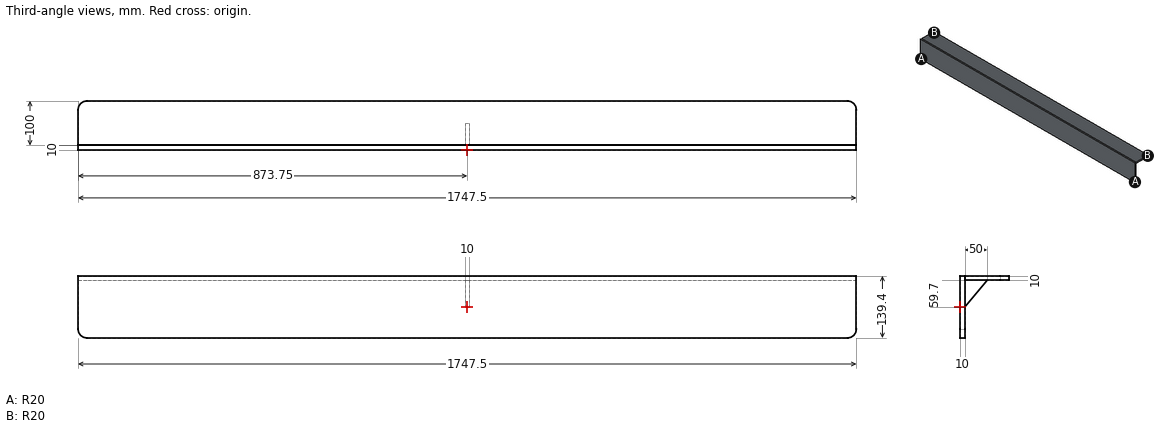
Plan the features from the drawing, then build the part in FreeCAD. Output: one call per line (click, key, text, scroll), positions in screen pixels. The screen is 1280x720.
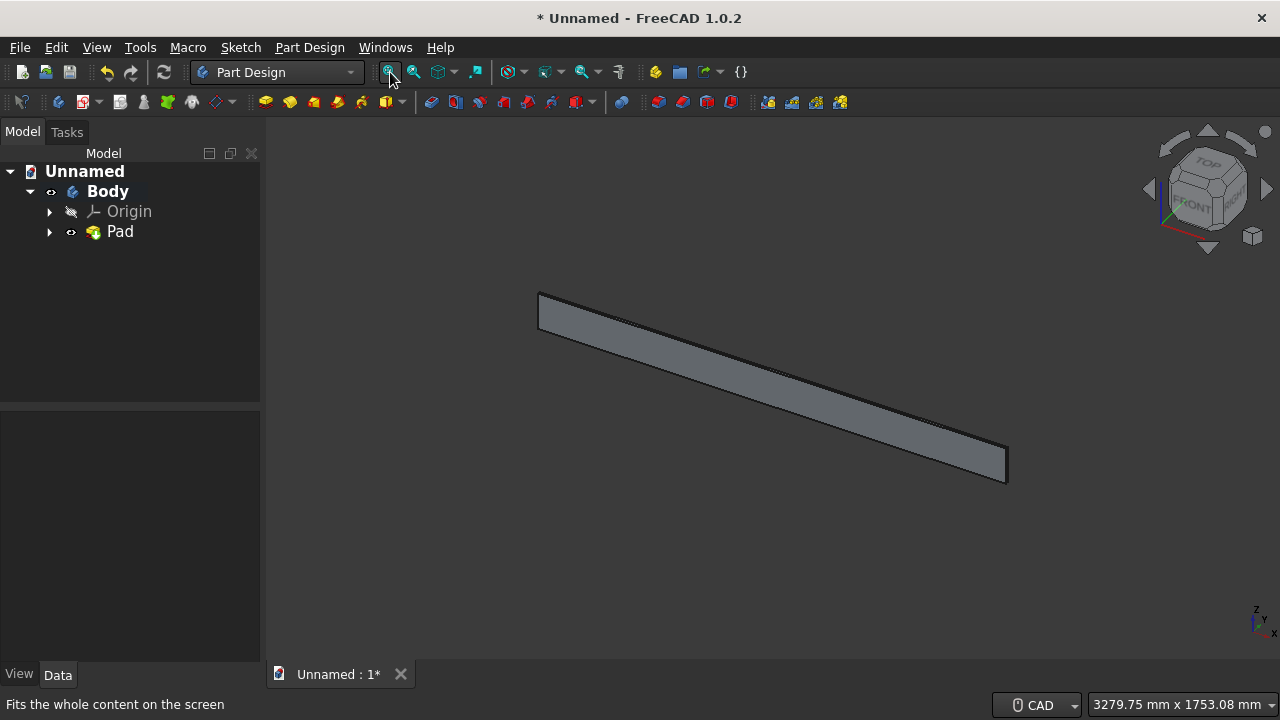
key(0)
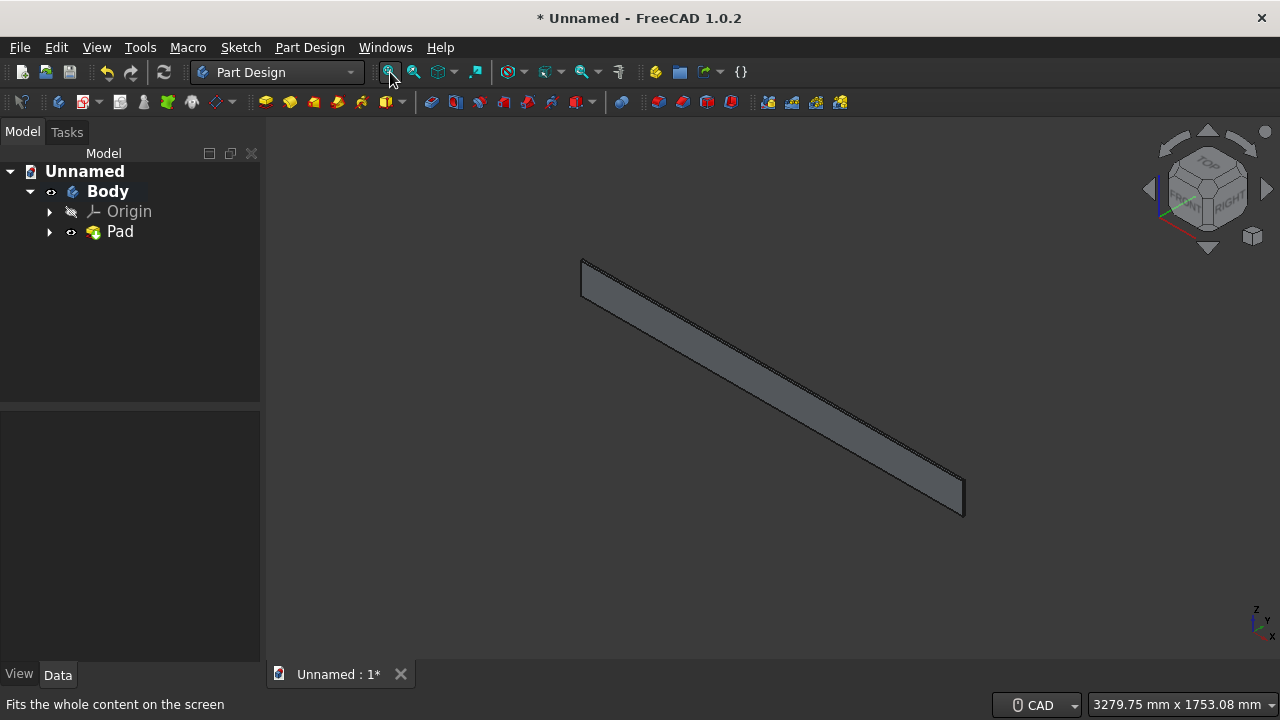
scroll(582, 294, up, 13)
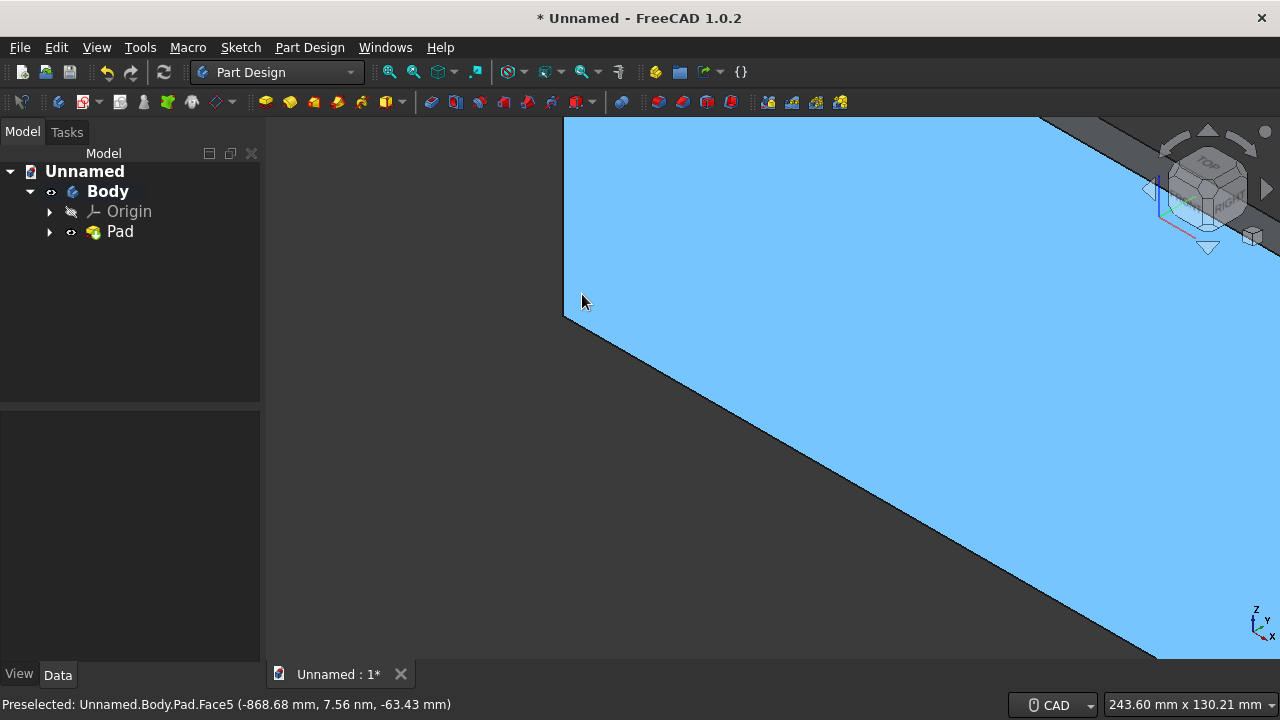
click(390, 72)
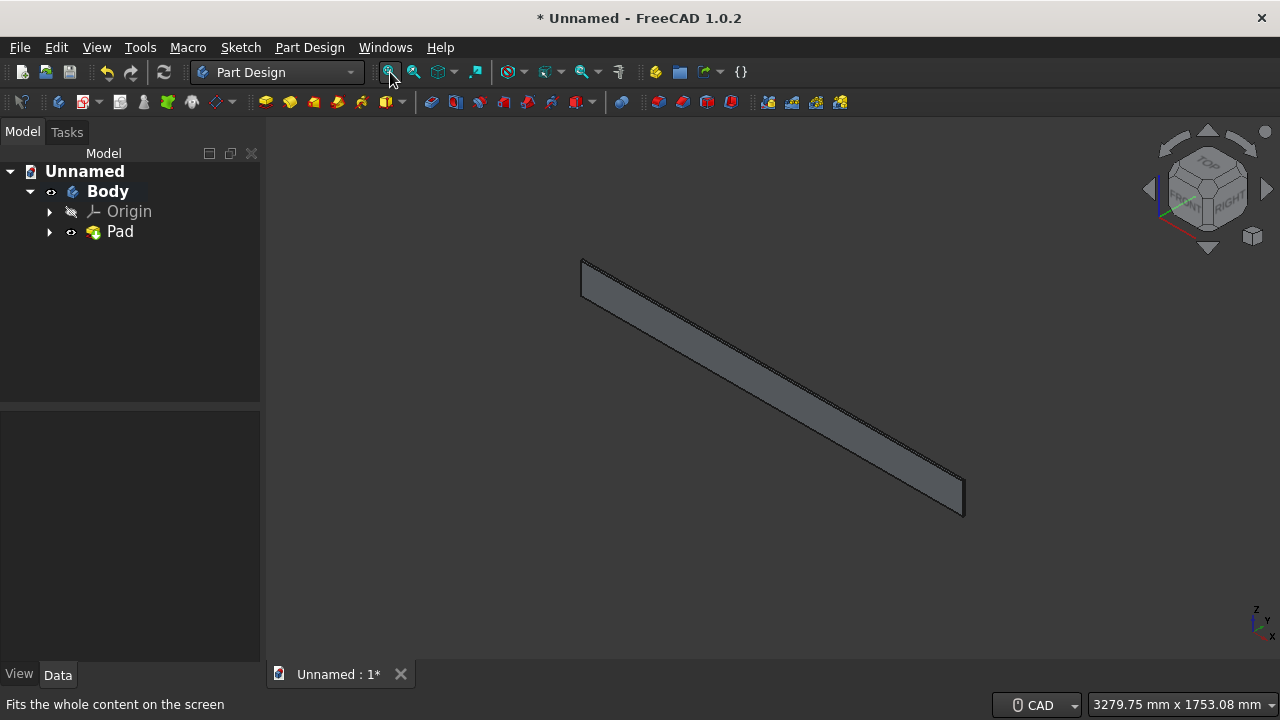
key(2)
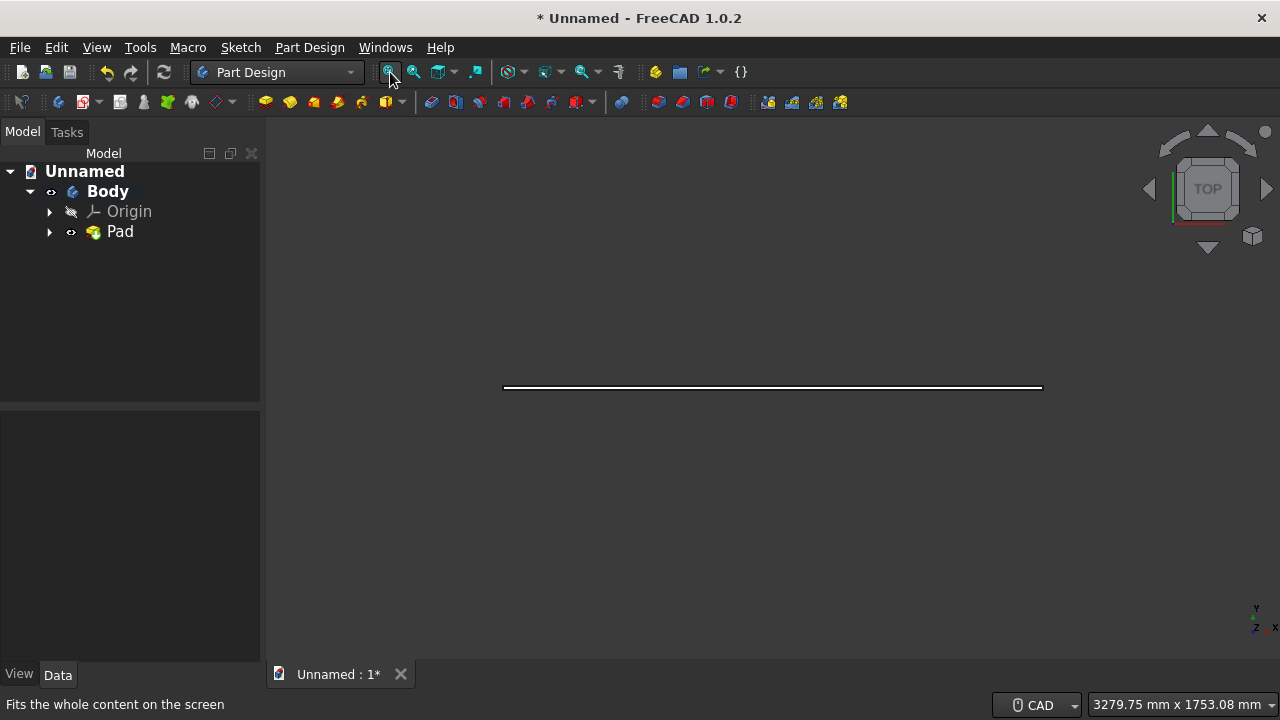
scroll(503, 387, up, 13)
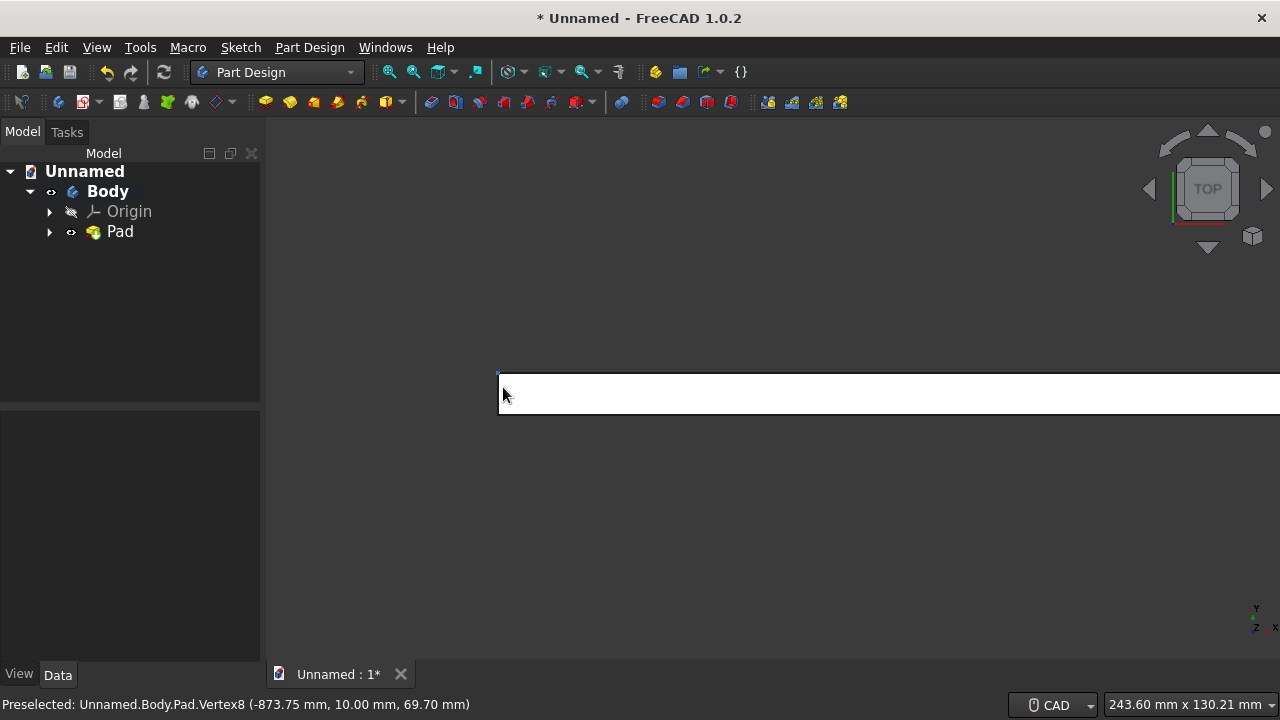
click(390, 72)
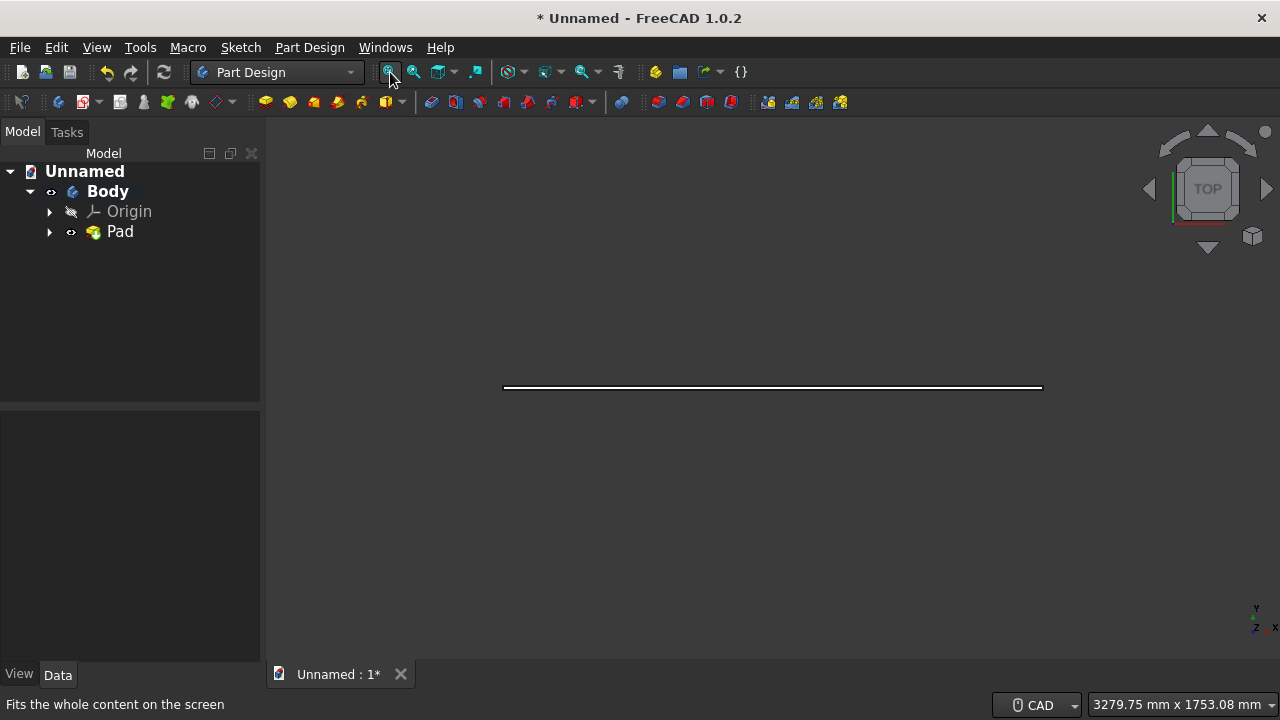
key(1)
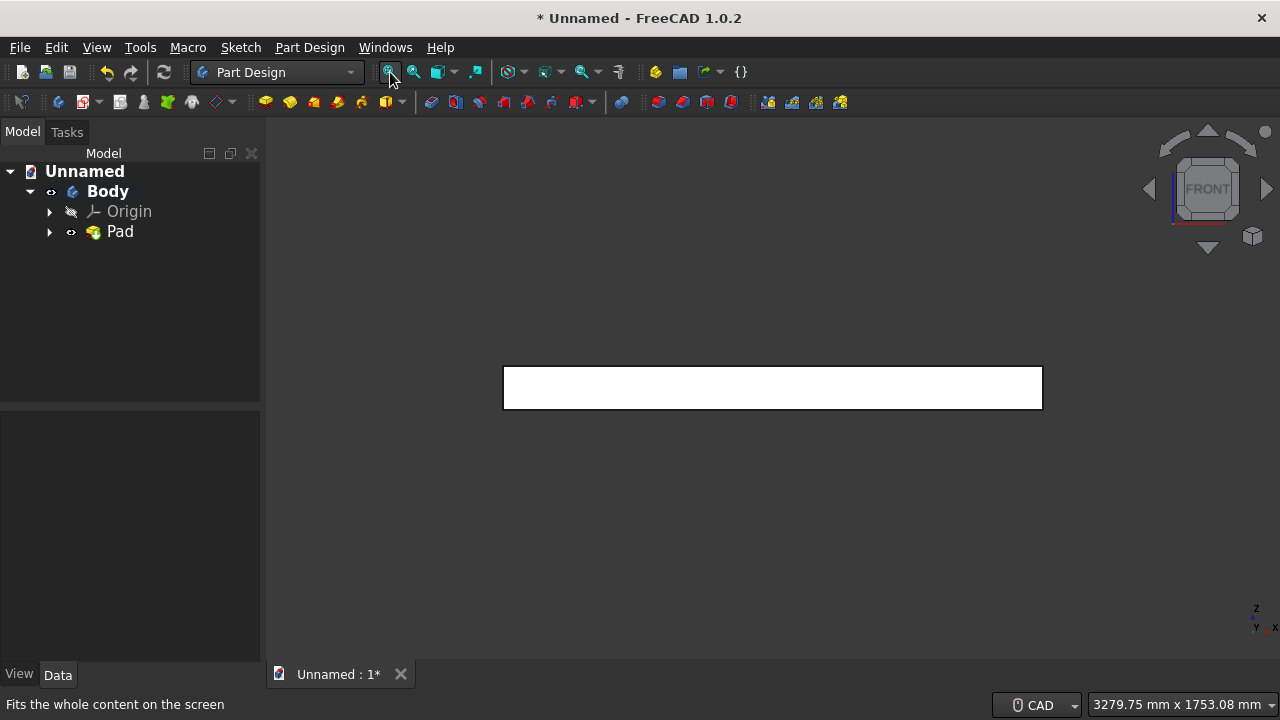
scroll(503, 409, up, 13)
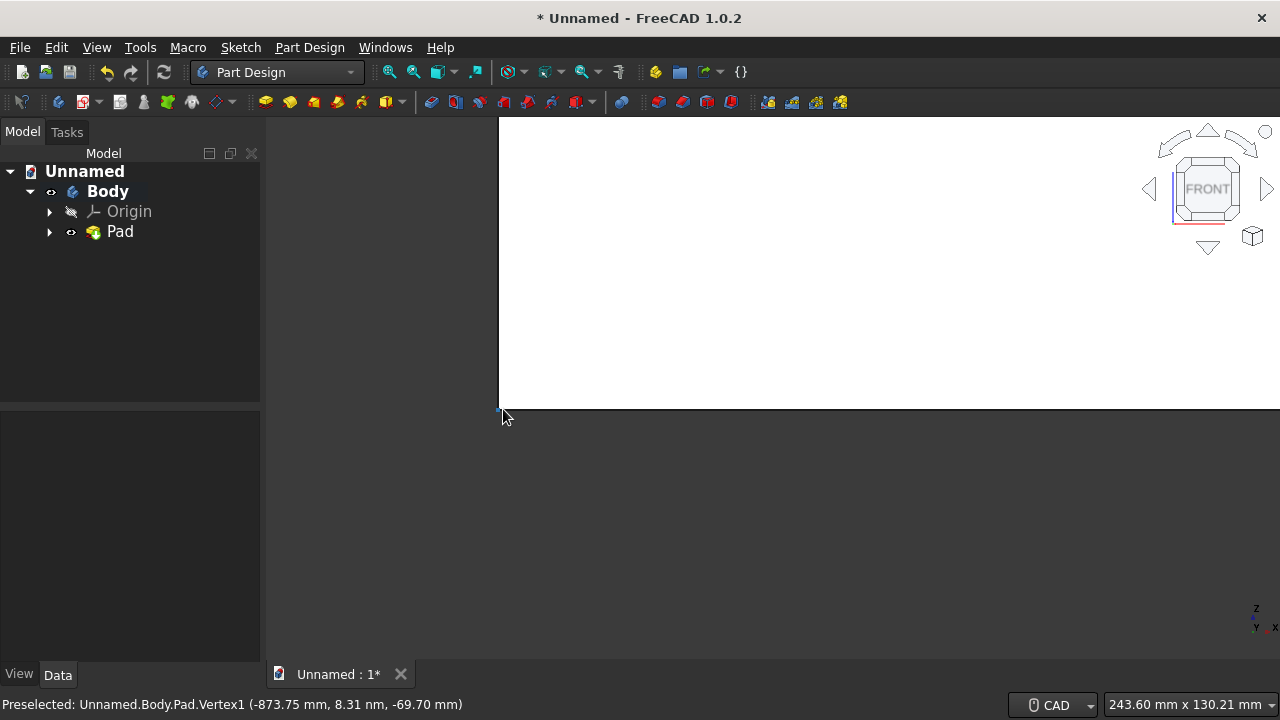
click(390, 72)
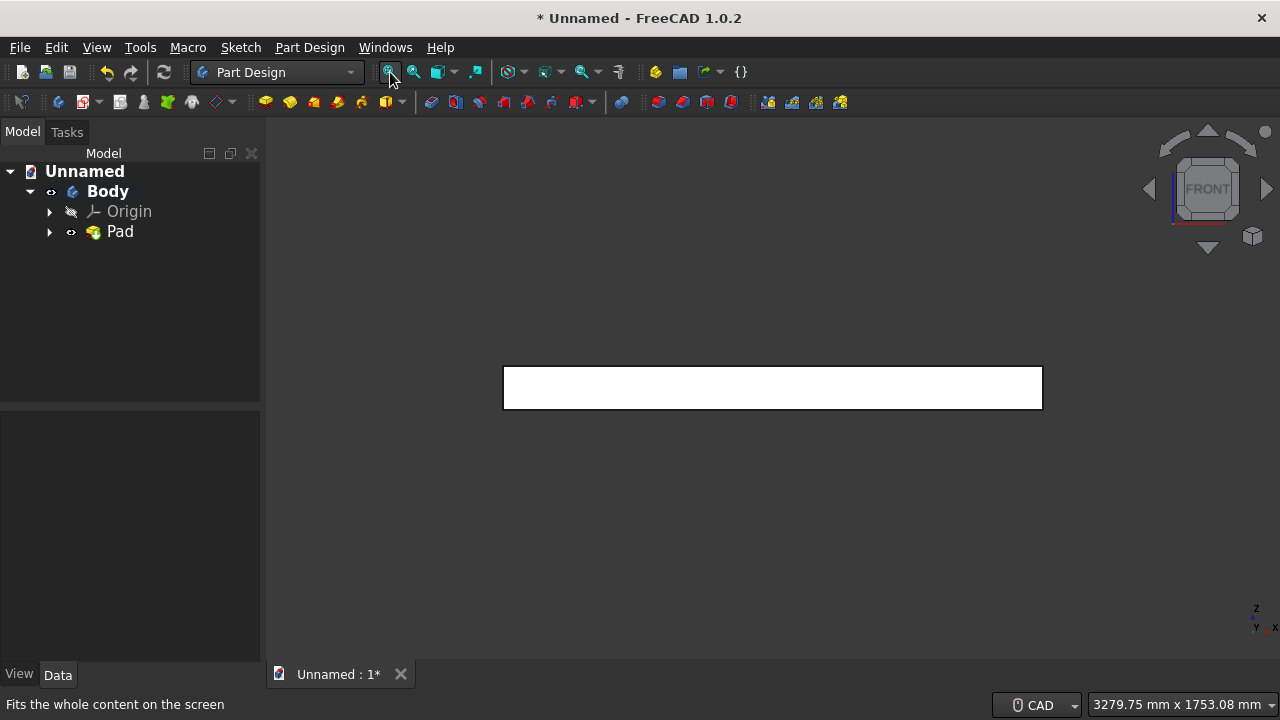
key(3)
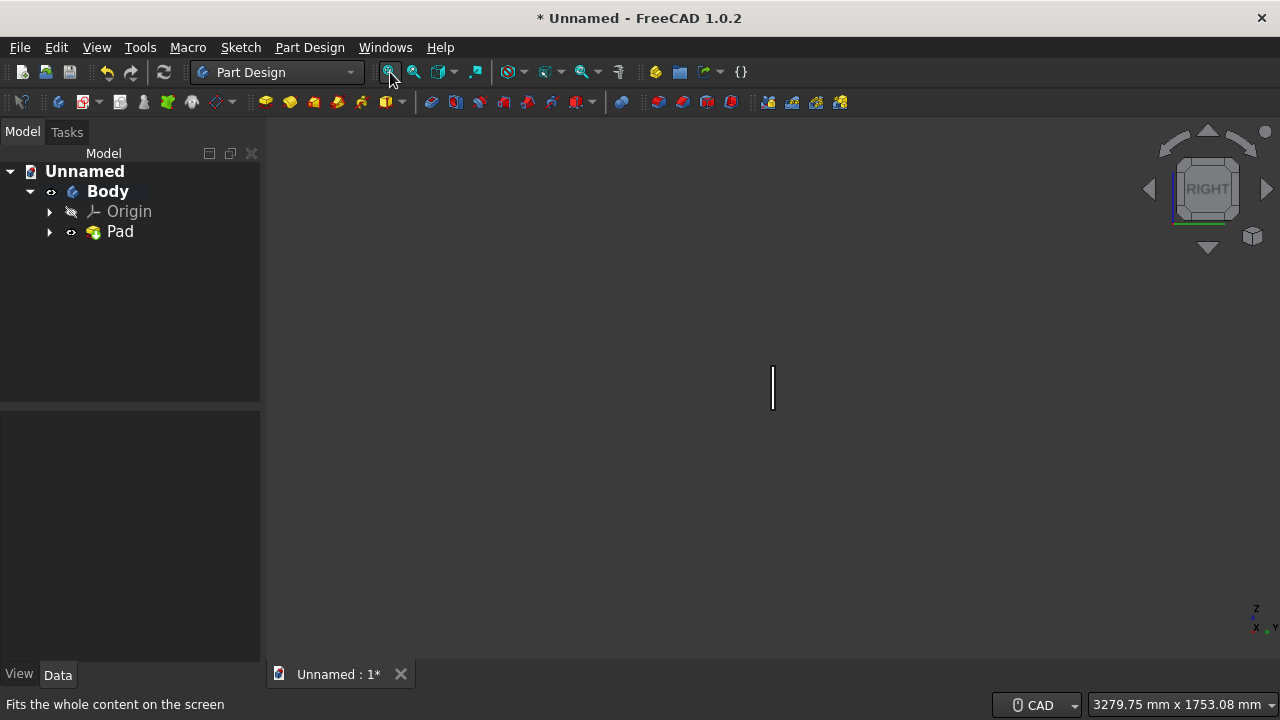
click(390, 72)